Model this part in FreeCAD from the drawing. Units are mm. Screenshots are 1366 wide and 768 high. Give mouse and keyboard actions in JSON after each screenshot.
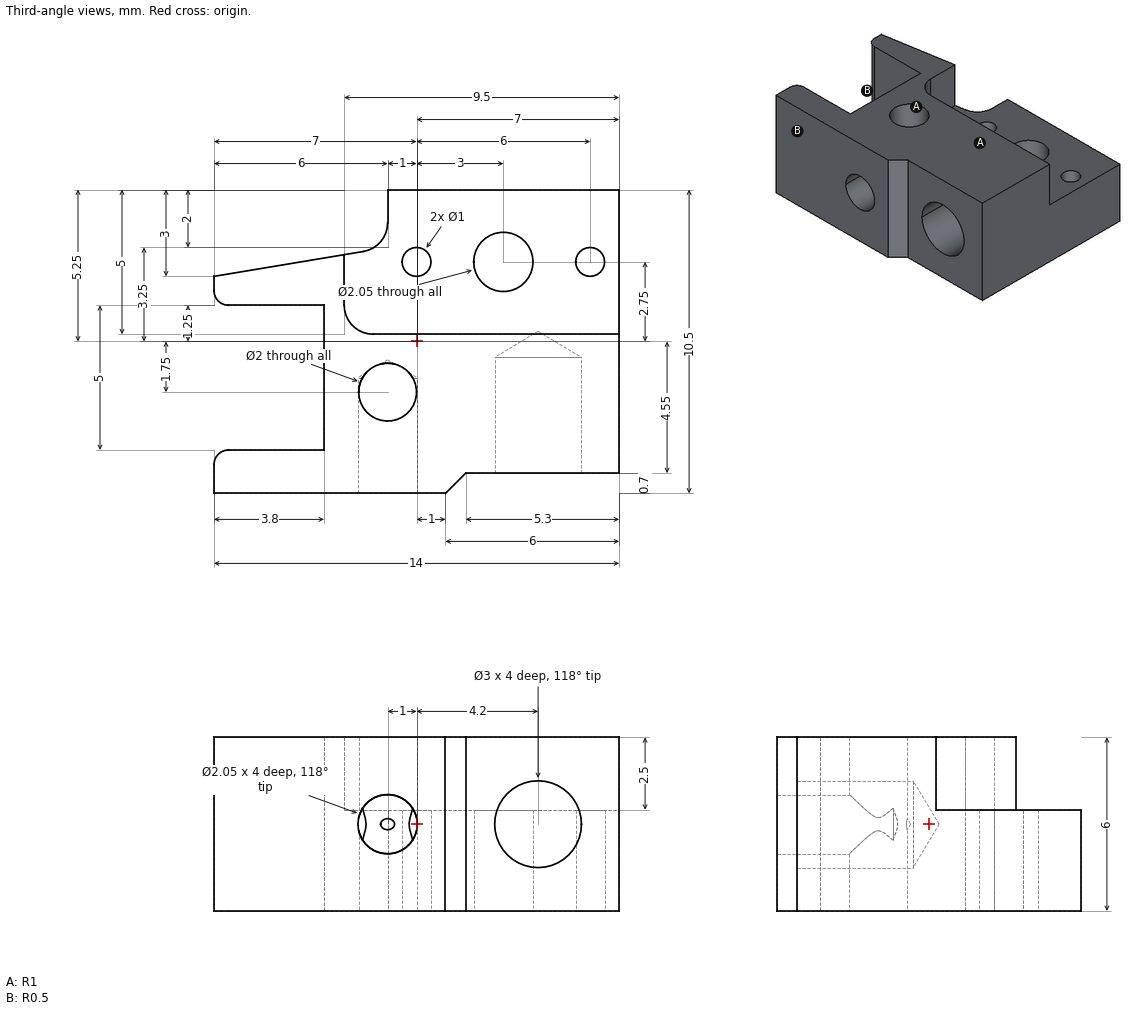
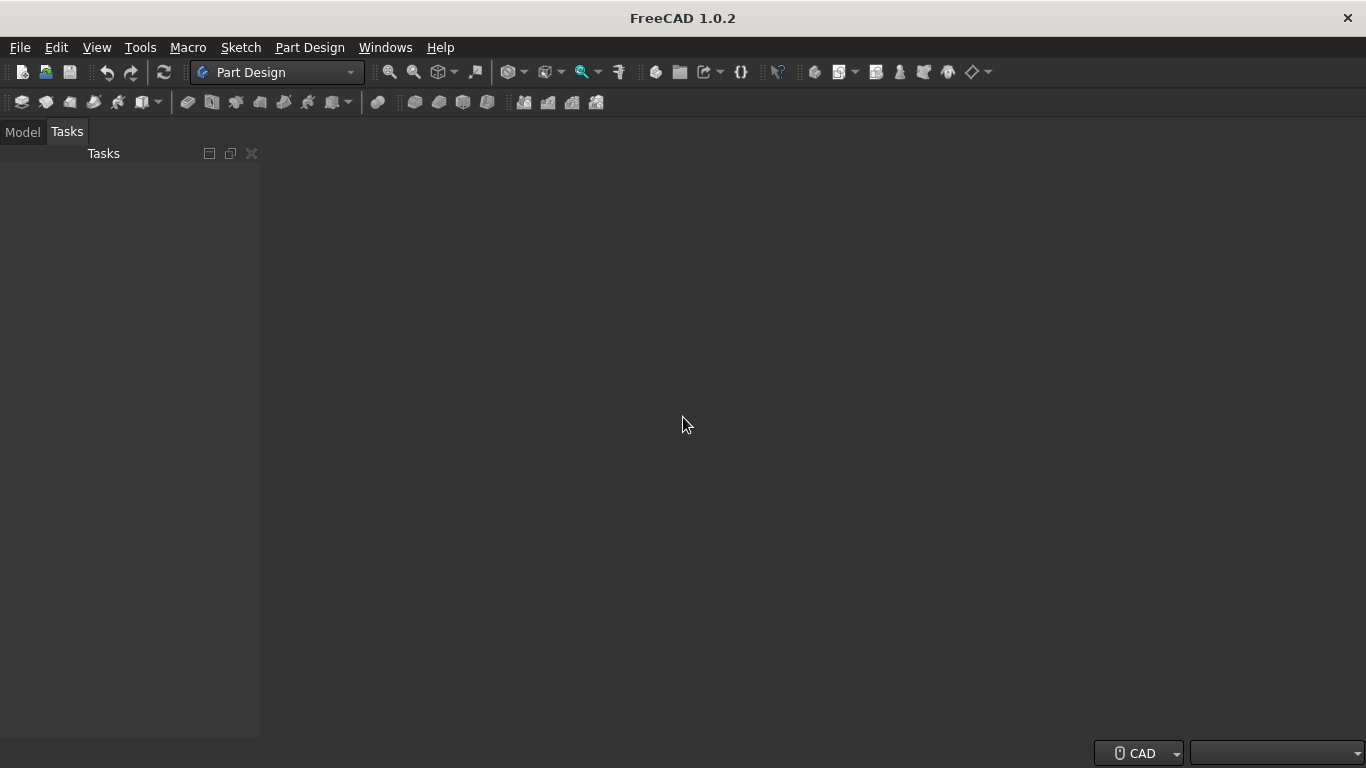
{"action": "left_click", "coordinate": [22, 72]}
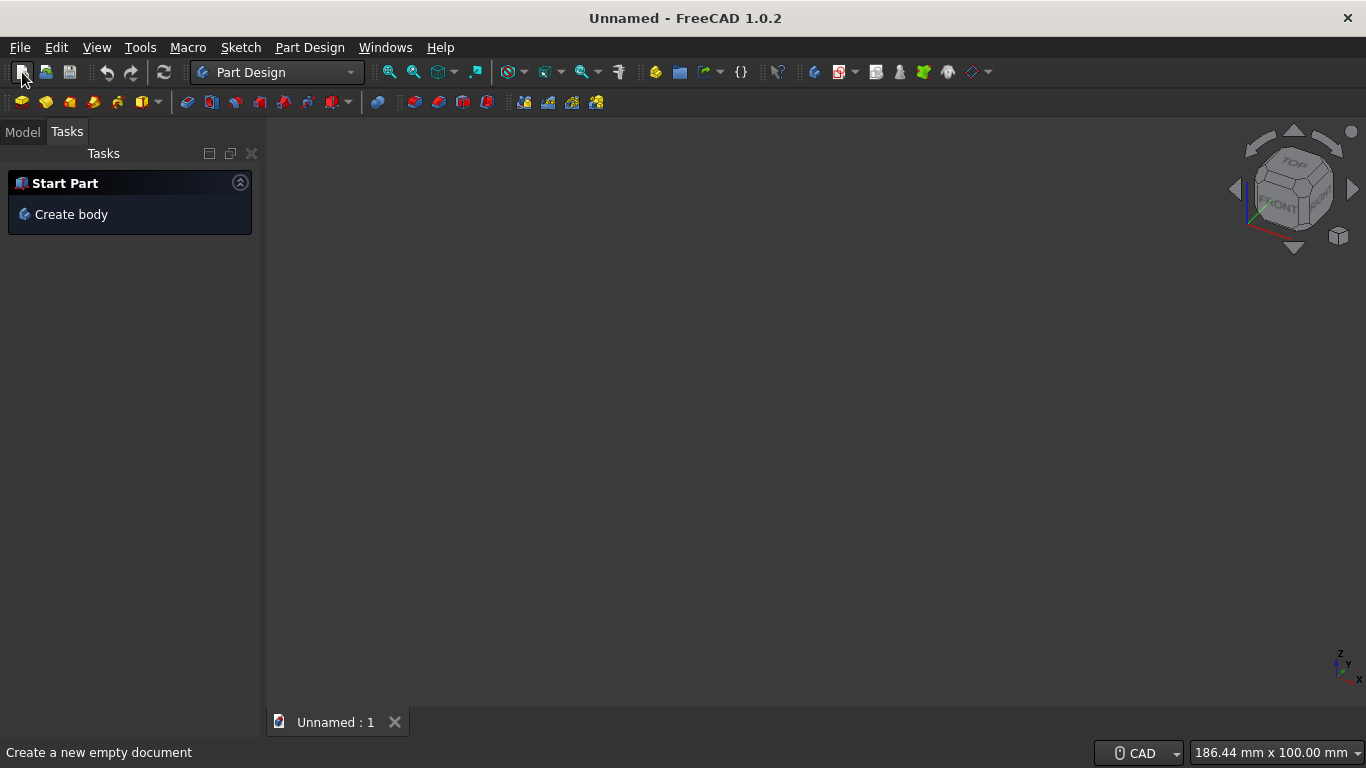
{"action": "left_click", "coordinate": [840, 72]}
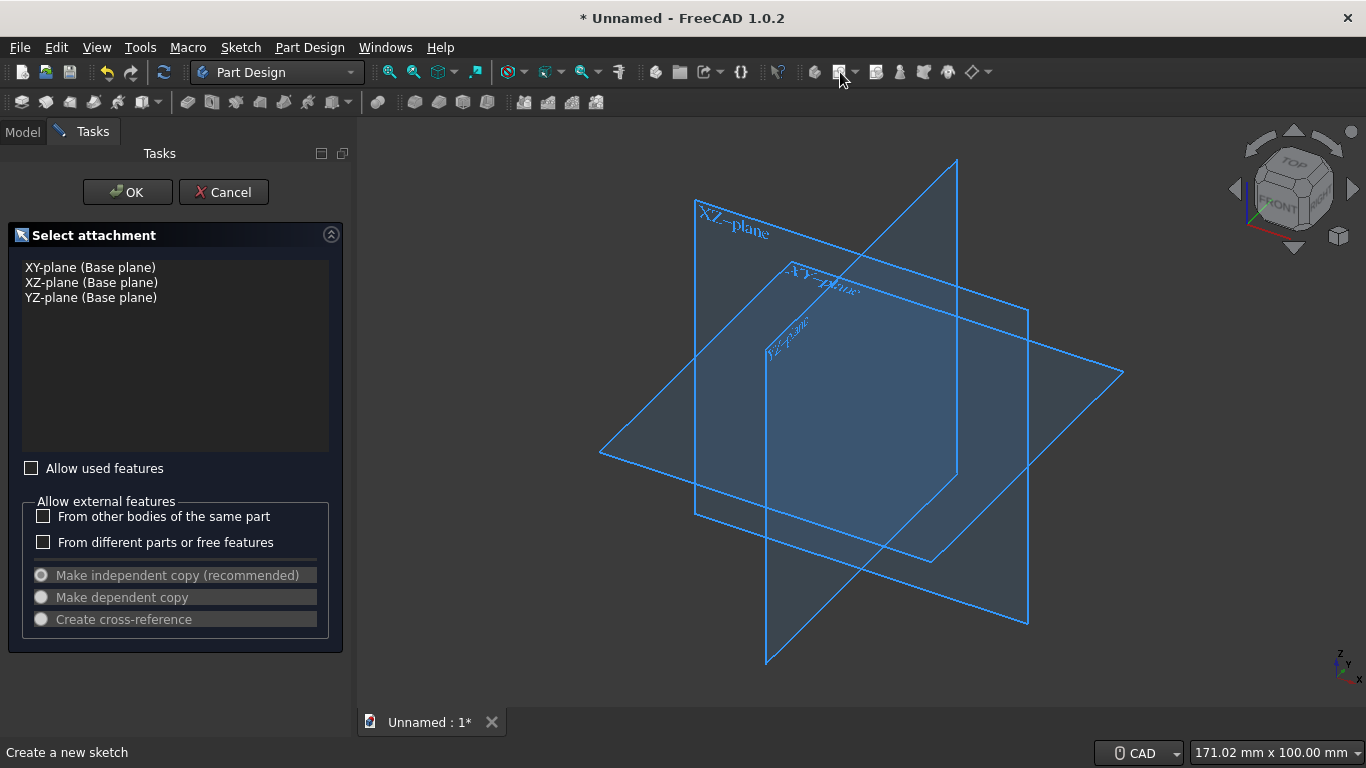
{"action": "left_click", "coordinate": [82, 268]}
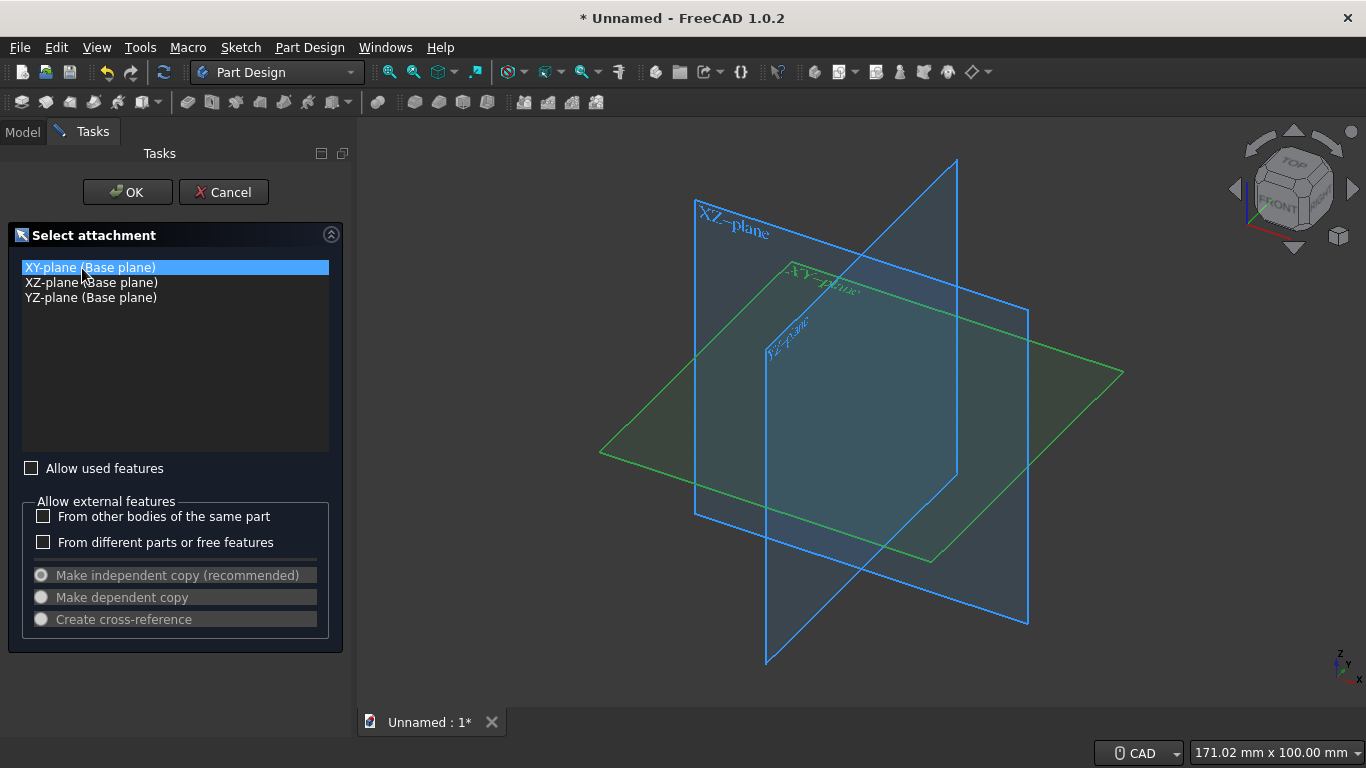
{"action": "left_click", "coordinate": [128, 192]}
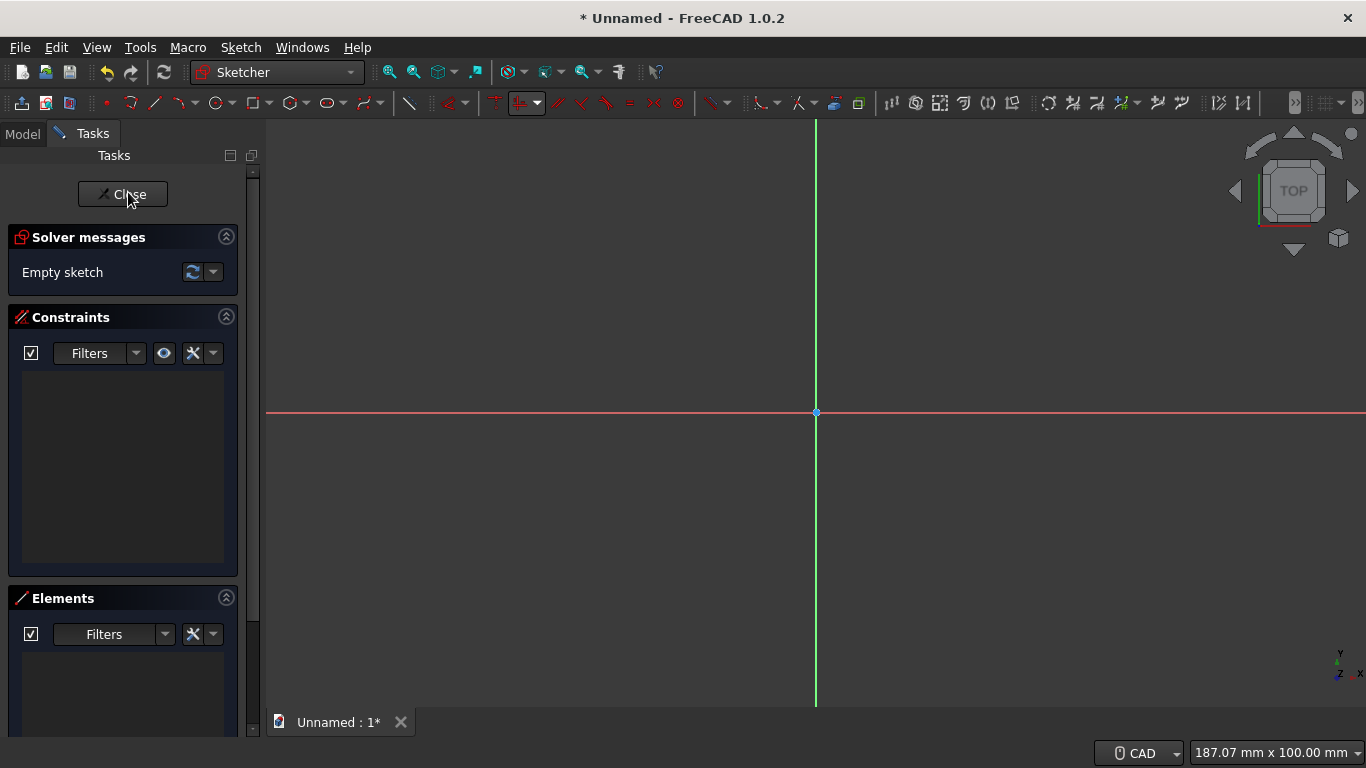
{"action": "scroll", "coordinate": [830, 413], "scroll_direction": "up", "scroll_amount": 9}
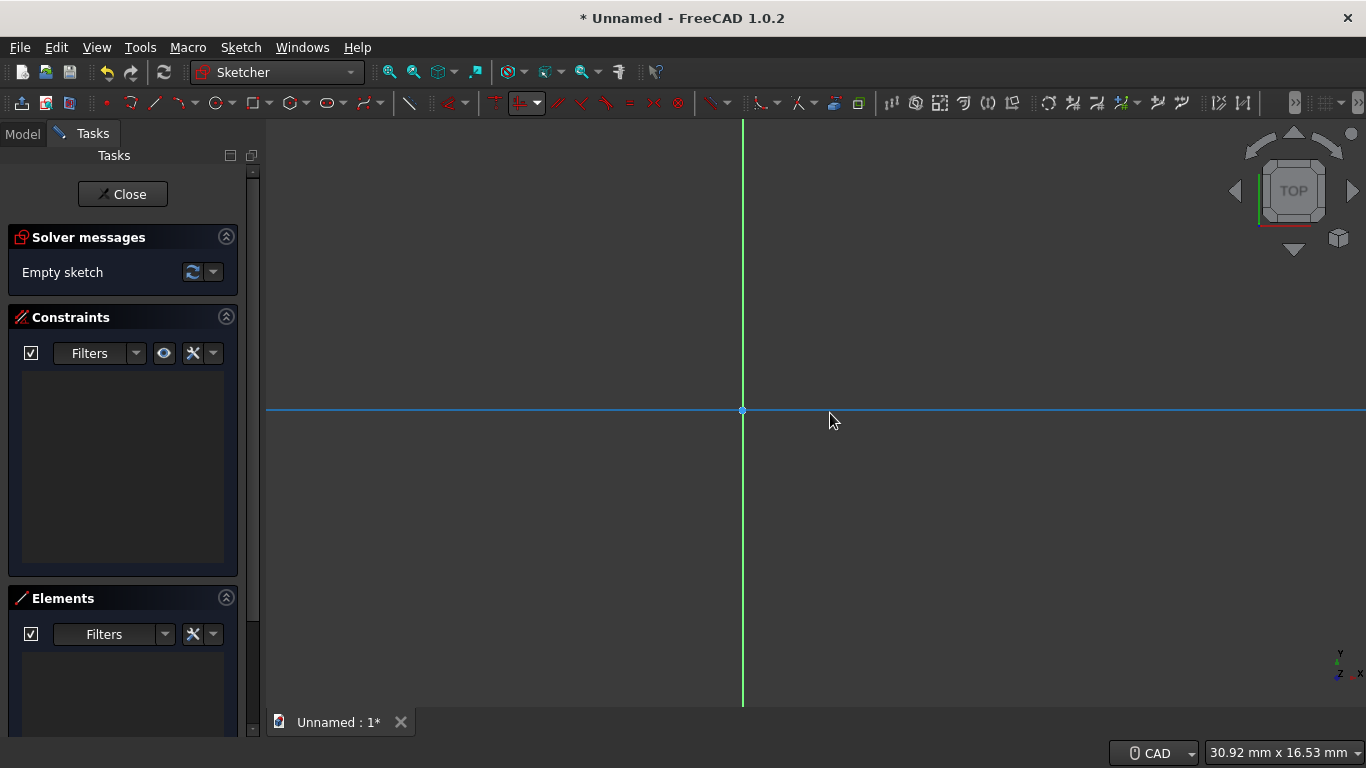
{"action": "left_click", "coordinate": [272, 104]}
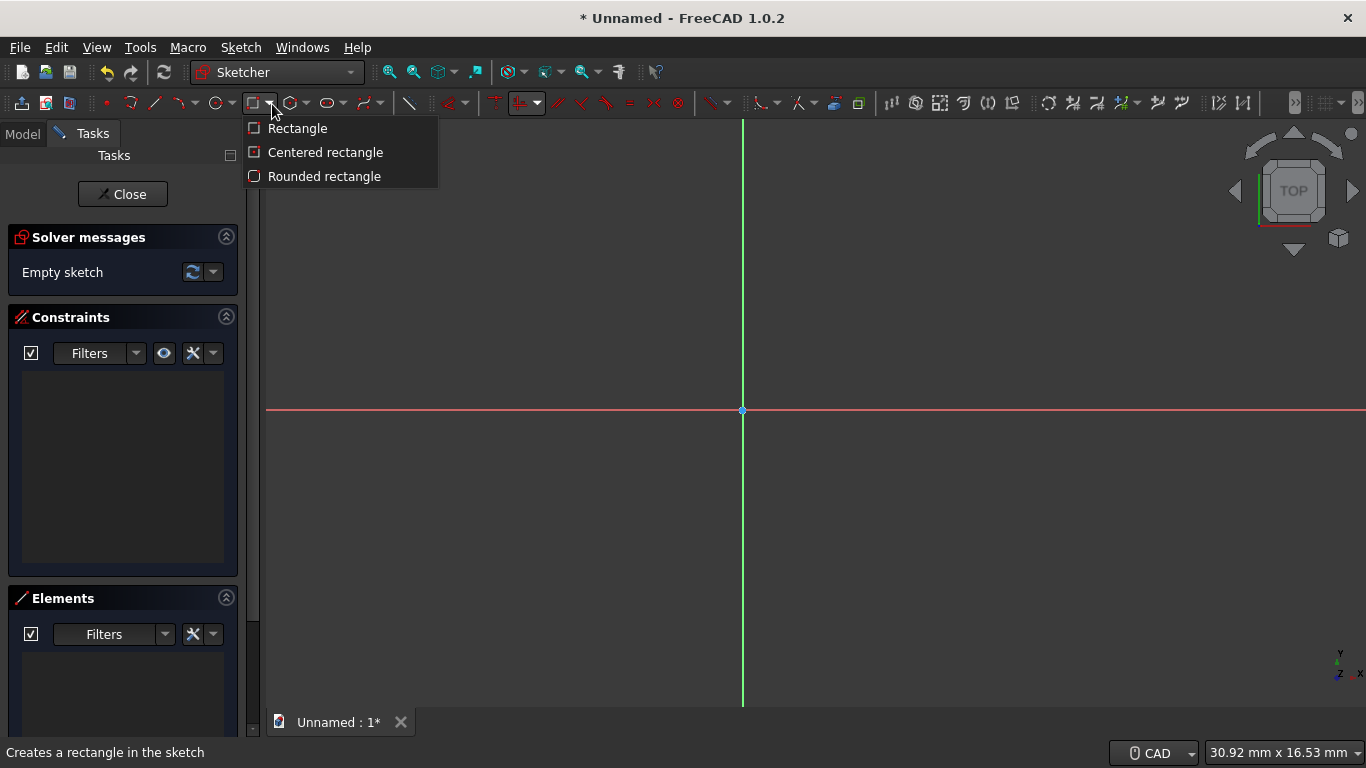
{"action": "left_click", "coordinate": [340, 152]}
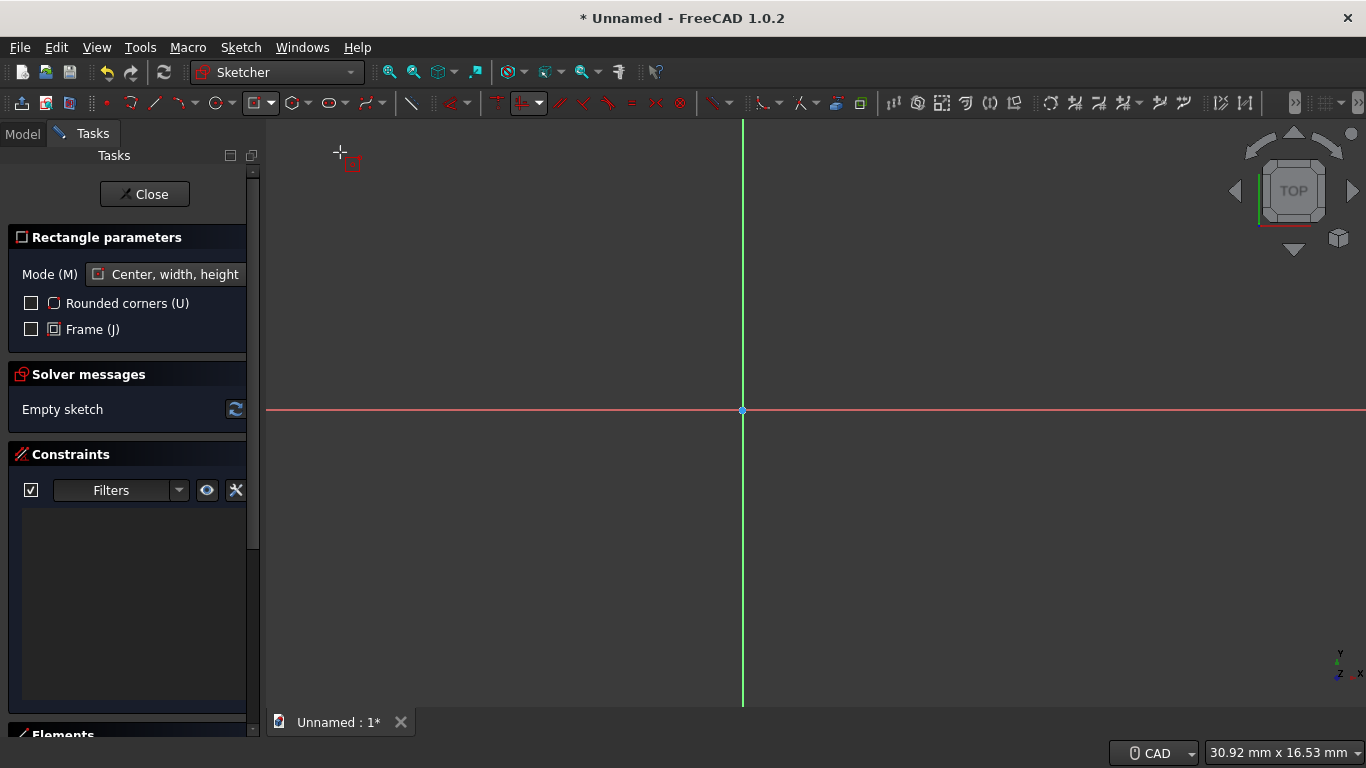
{"action": "left_click", "coordinate": [743, 410]}
{"action": "left_click", "coordinate": [992, 224]}
{"action": "key", "text": "Escape"}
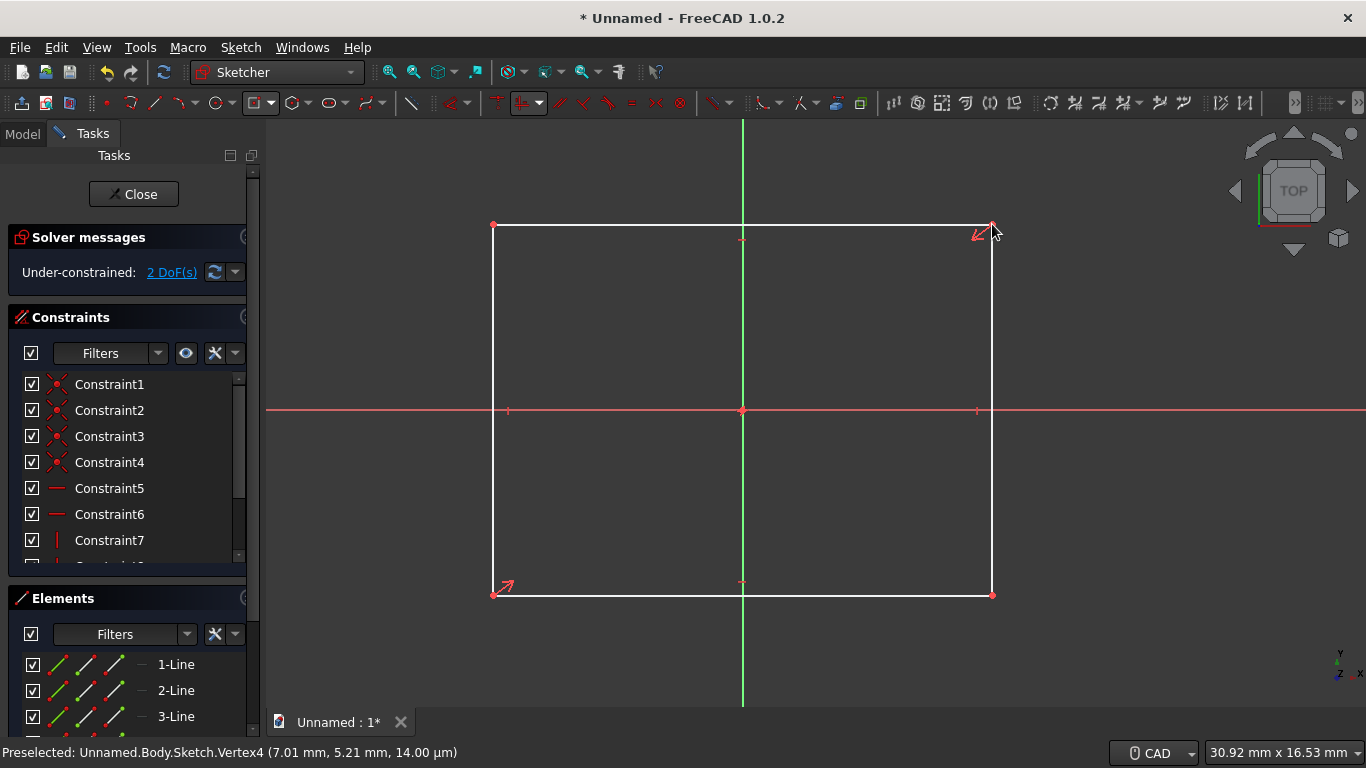
{"action": "left_click", "coordinate": [450, 104]}